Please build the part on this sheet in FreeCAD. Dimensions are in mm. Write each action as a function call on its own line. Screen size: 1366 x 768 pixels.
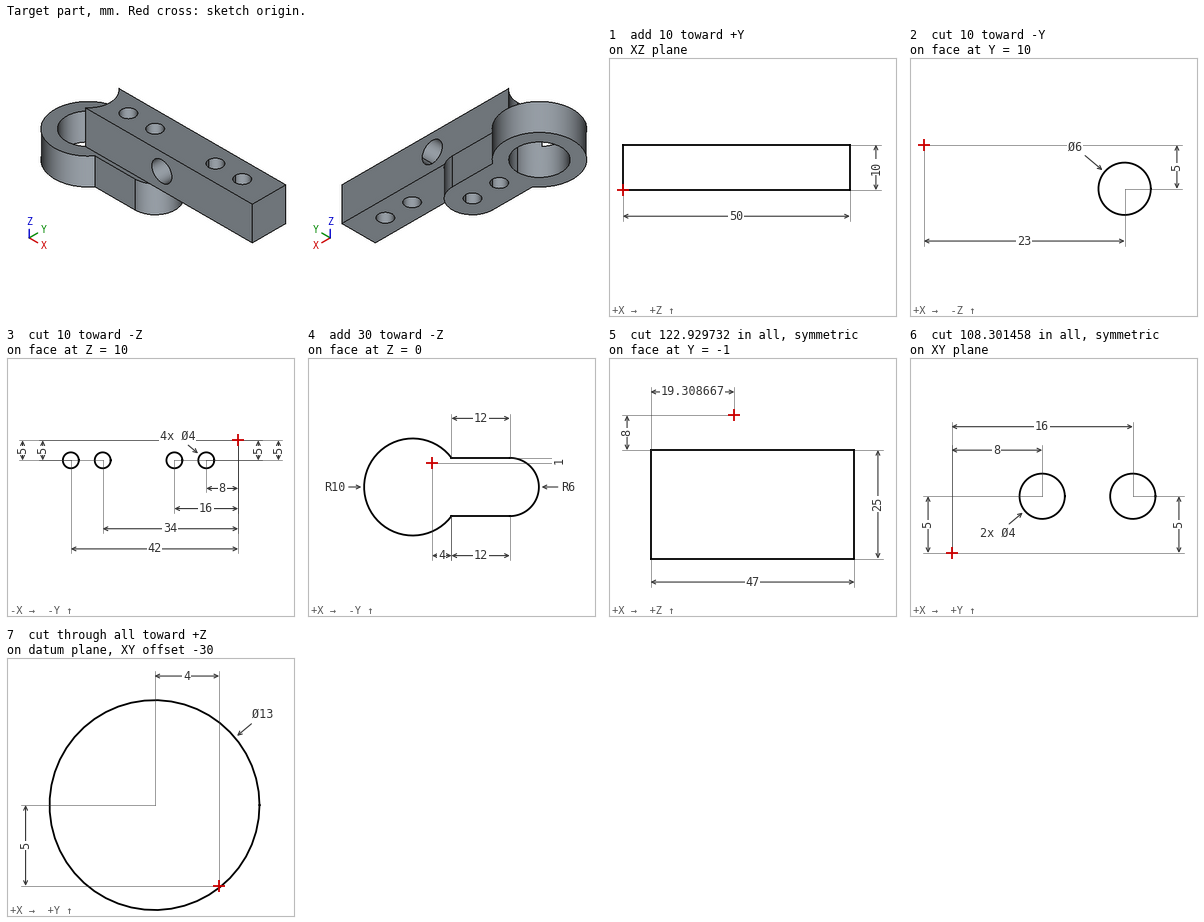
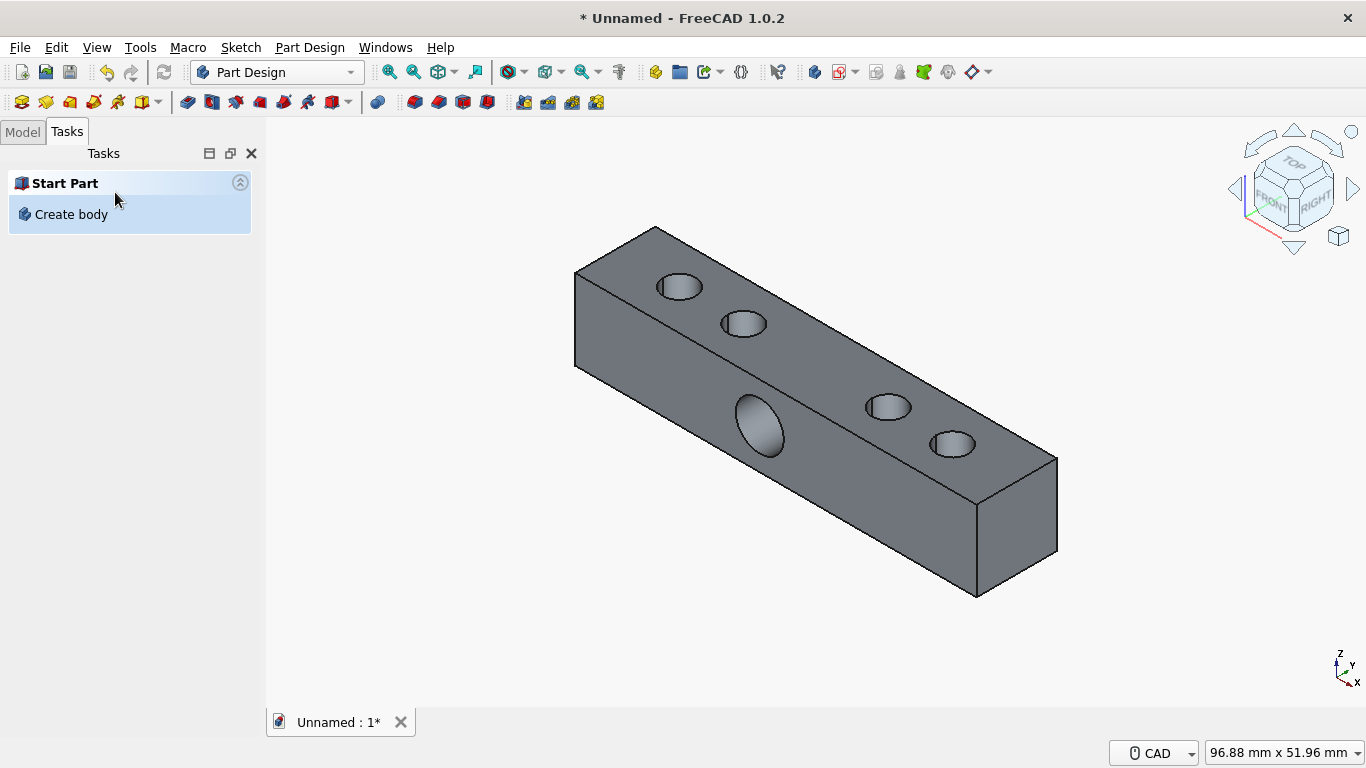
key(5)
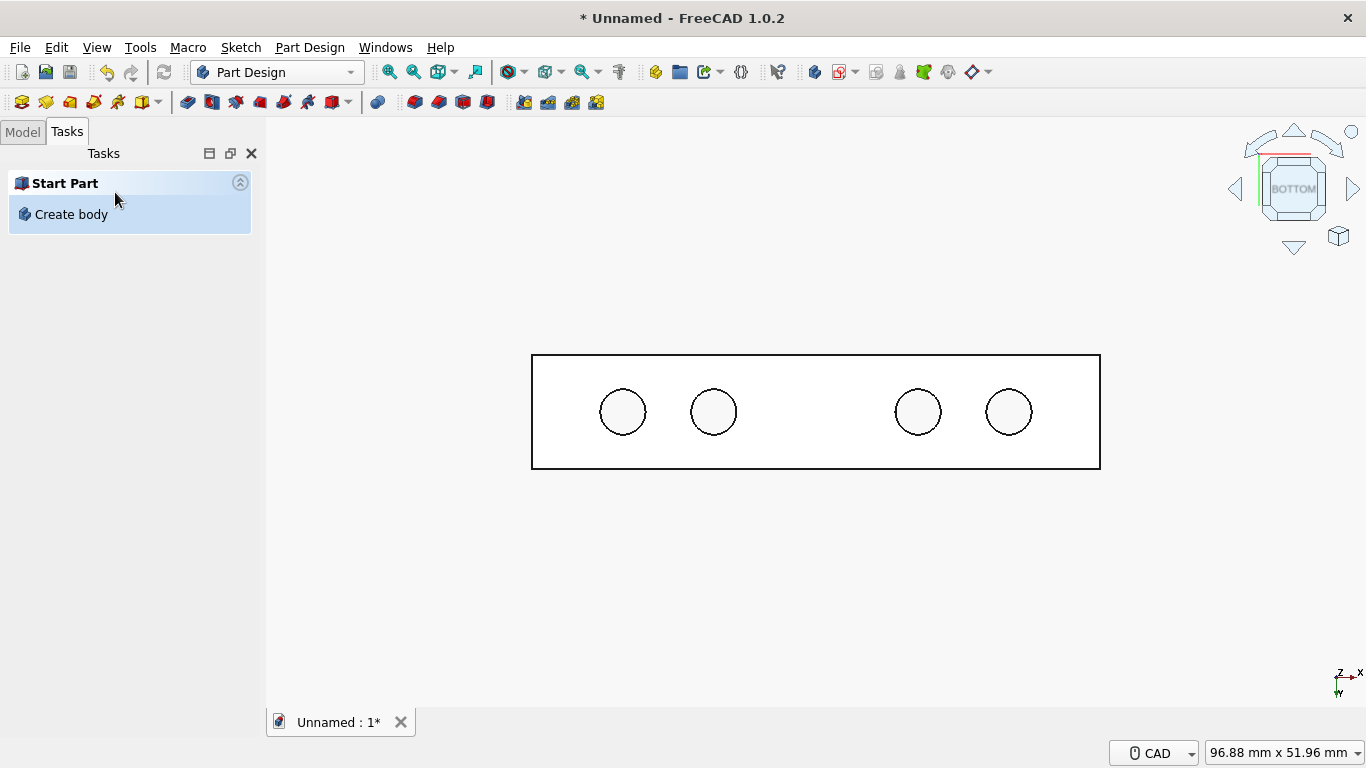
click(816, 411)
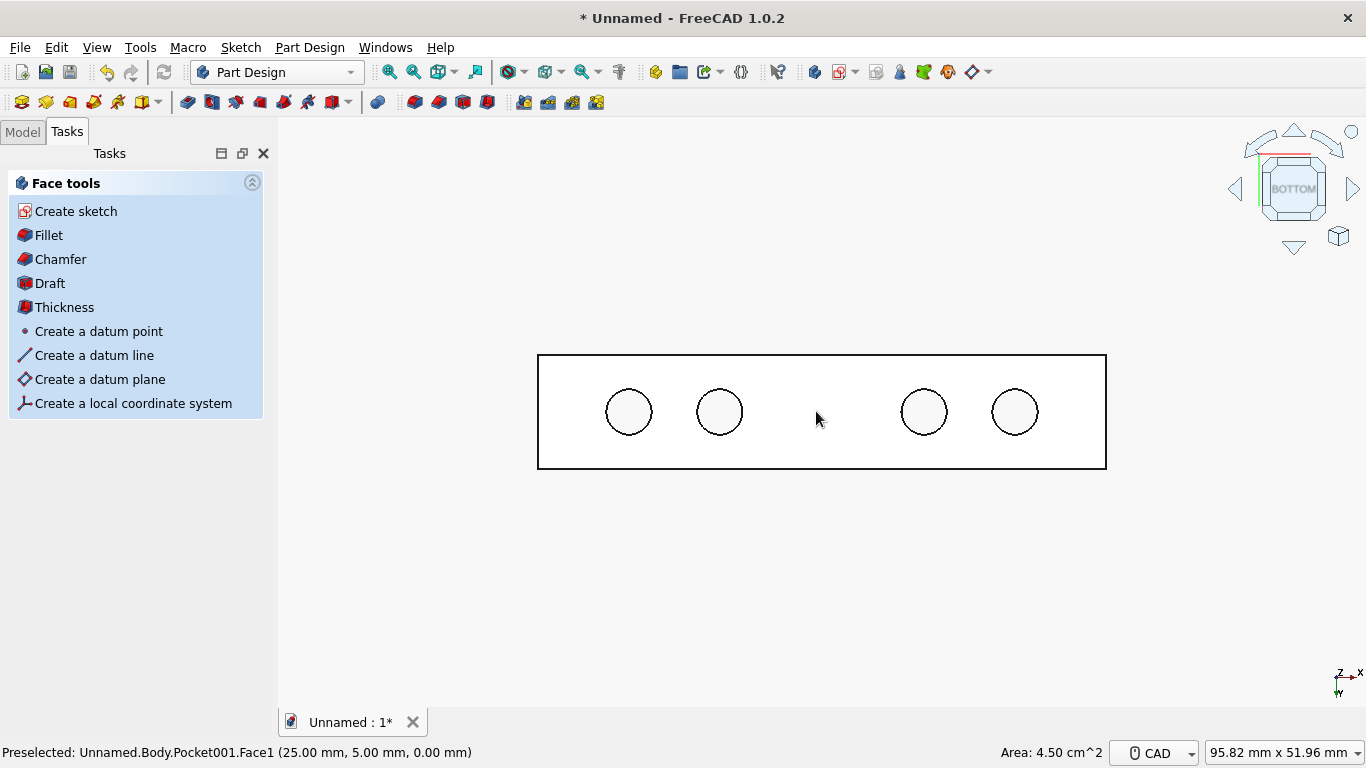
click(840, 72)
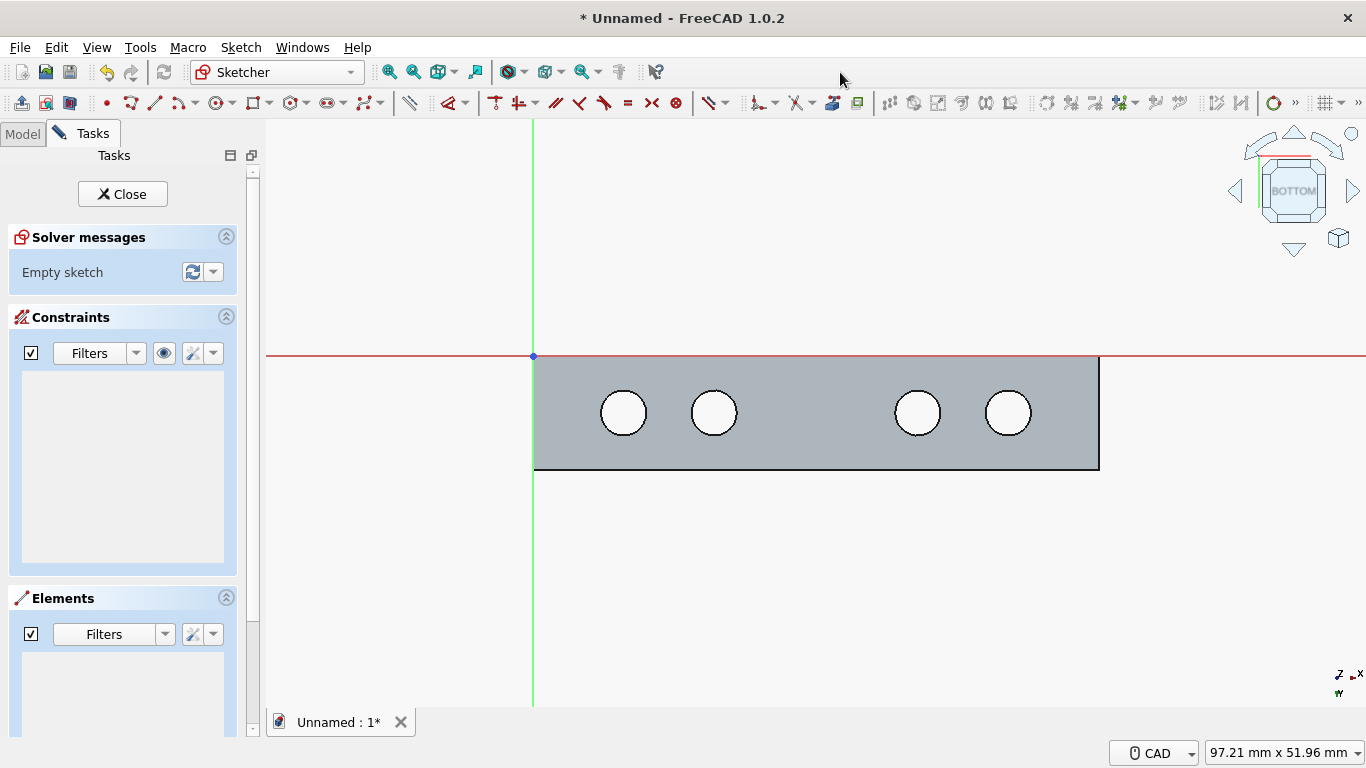
scroll(294, 413, up, 2)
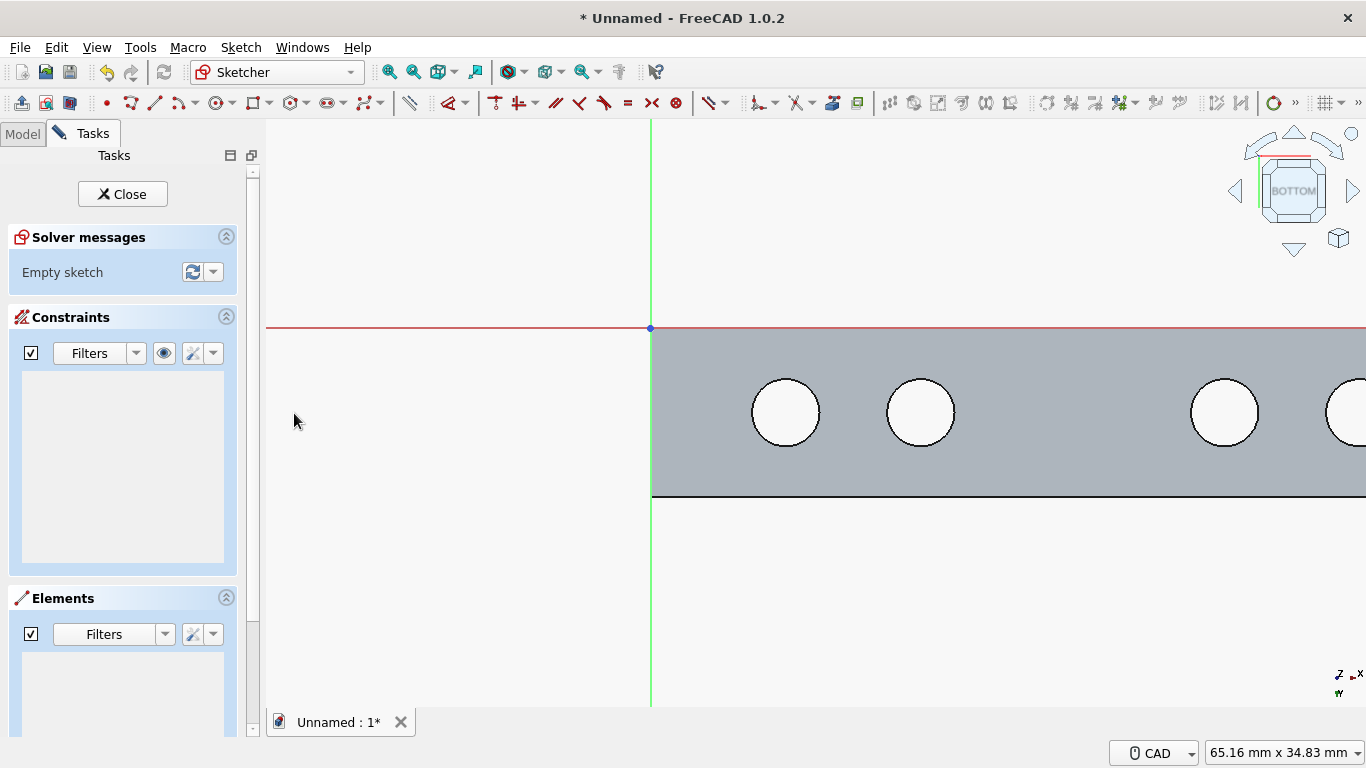
click(156, 104)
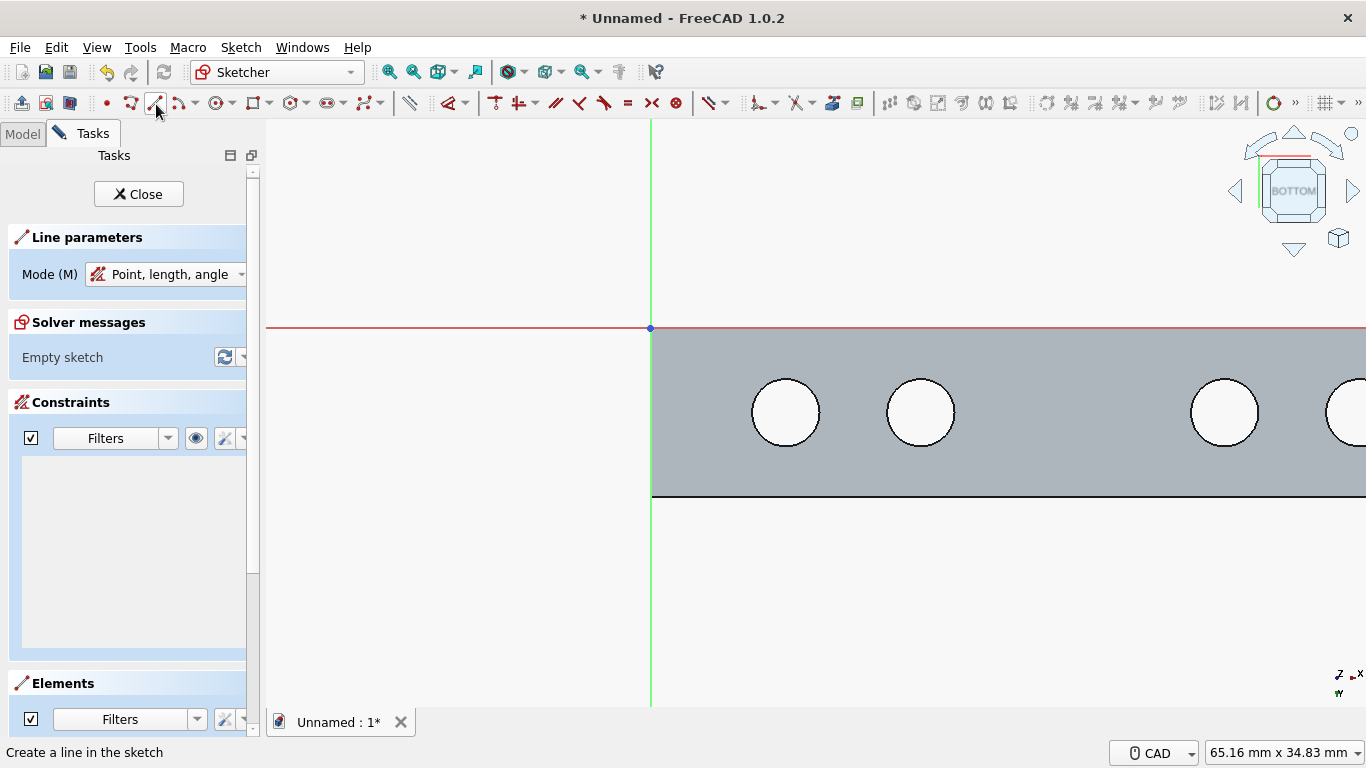
click(718, 514)
click(921, 514)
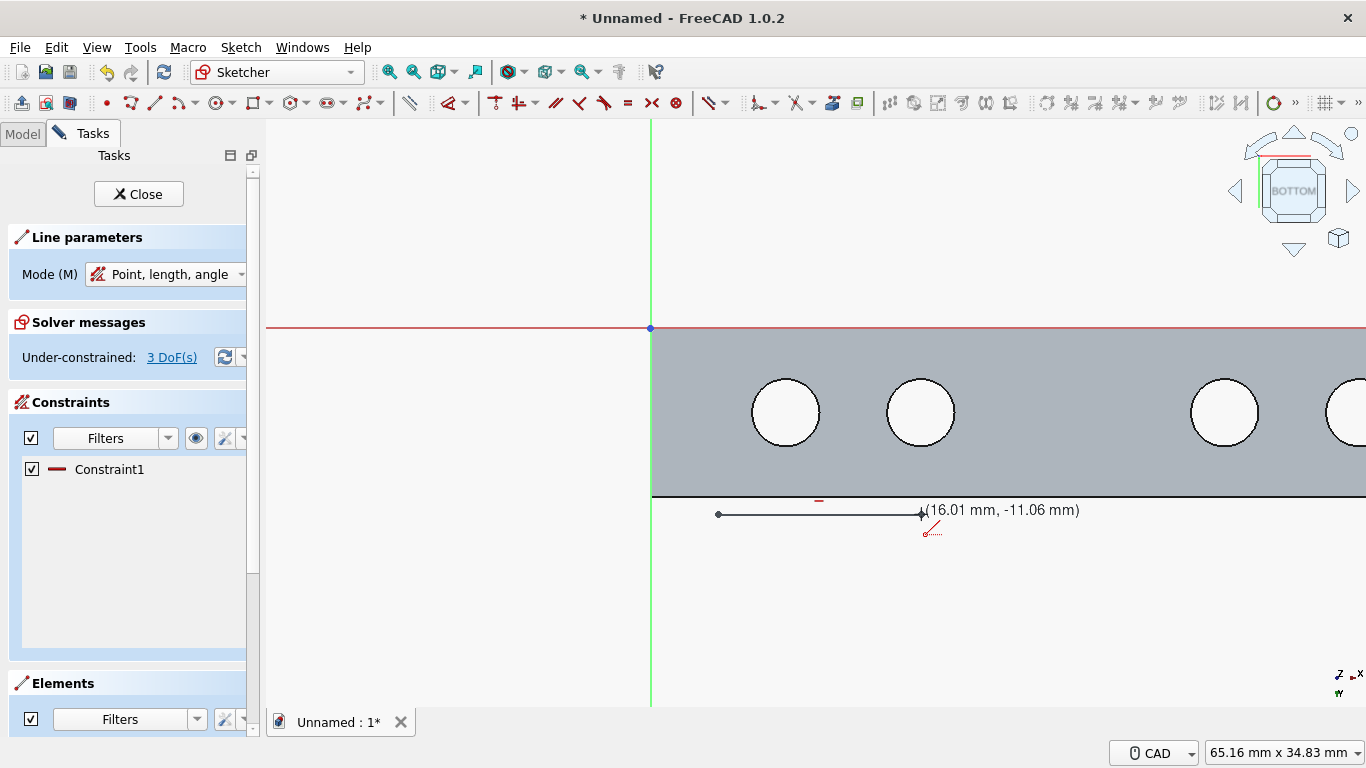
click(921, 311)
click(718, 311)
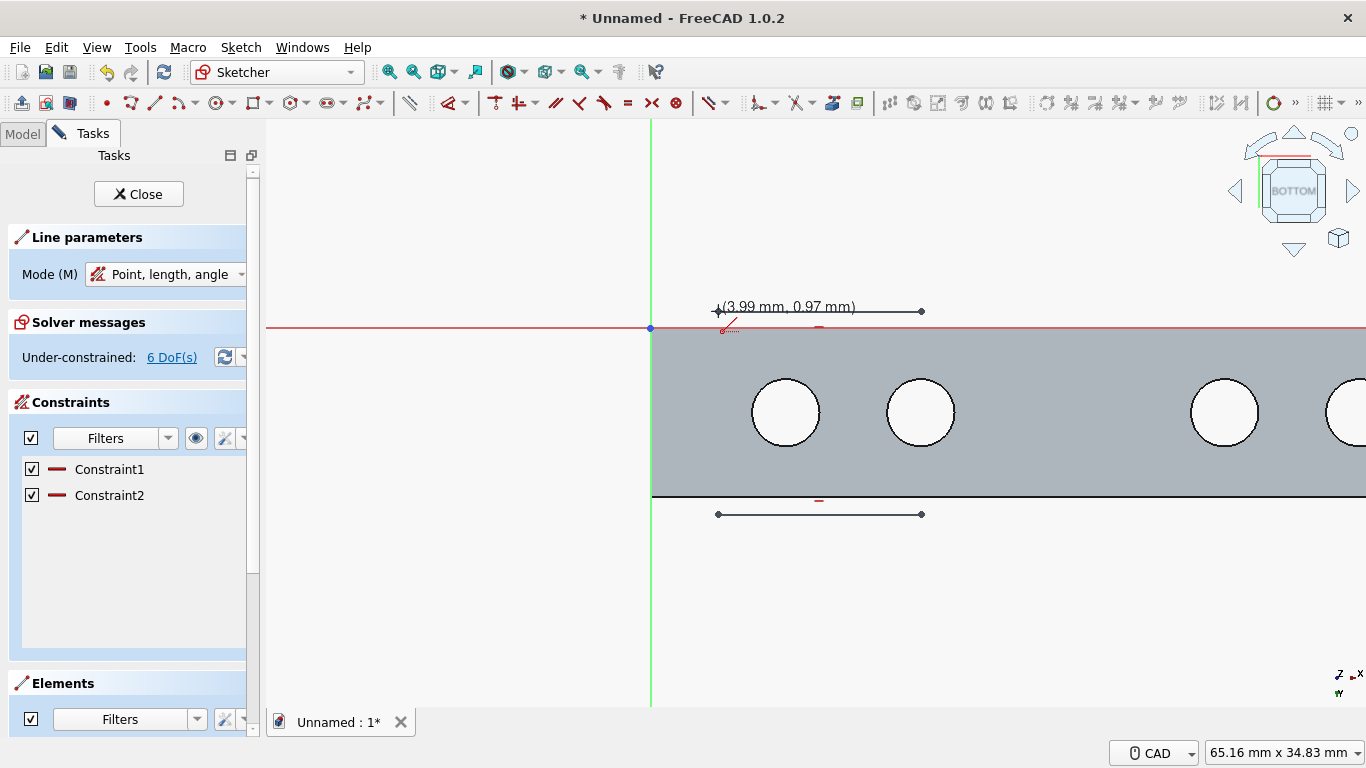
click(198, 104)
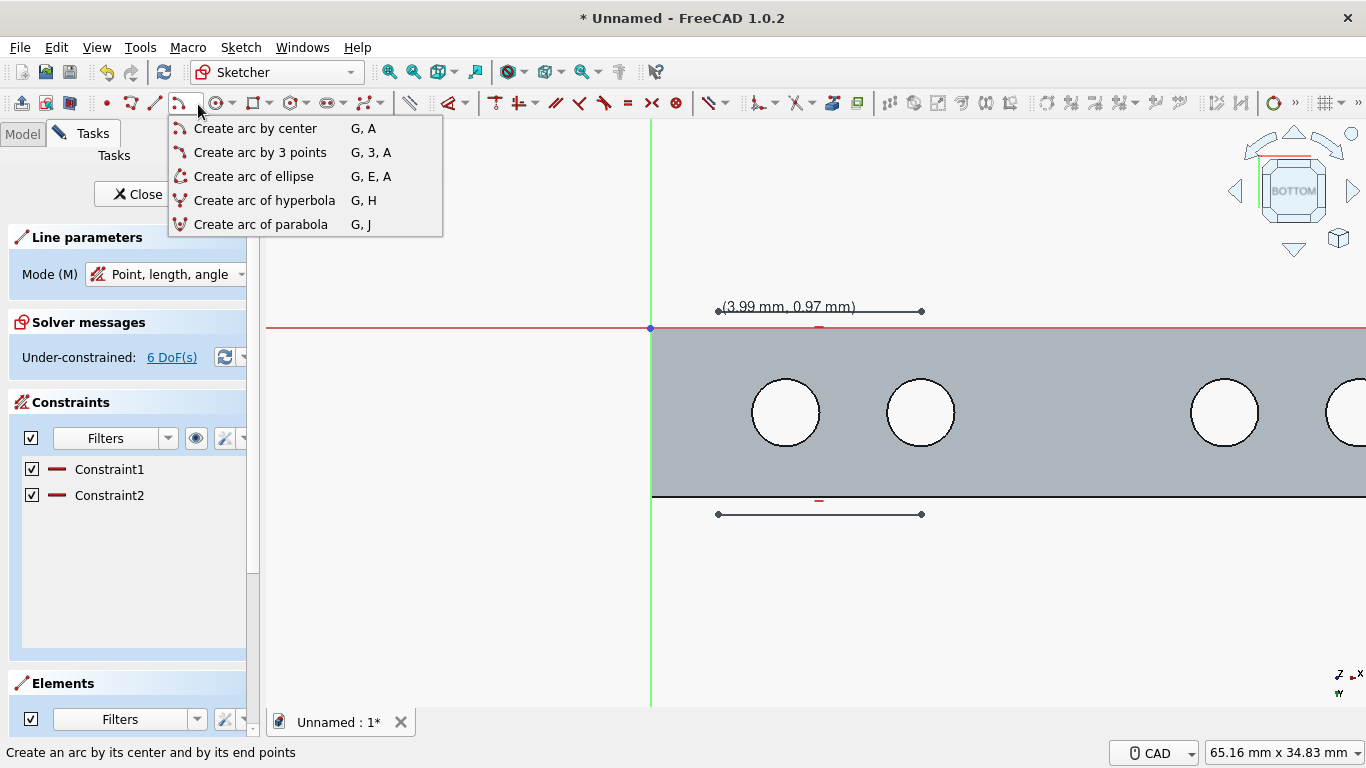
click(306, 152)